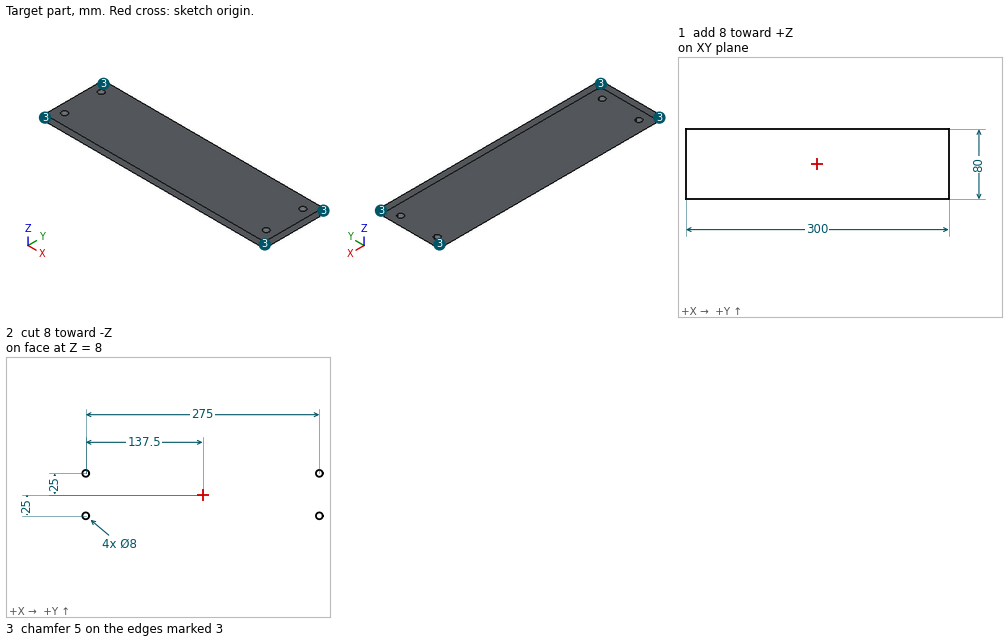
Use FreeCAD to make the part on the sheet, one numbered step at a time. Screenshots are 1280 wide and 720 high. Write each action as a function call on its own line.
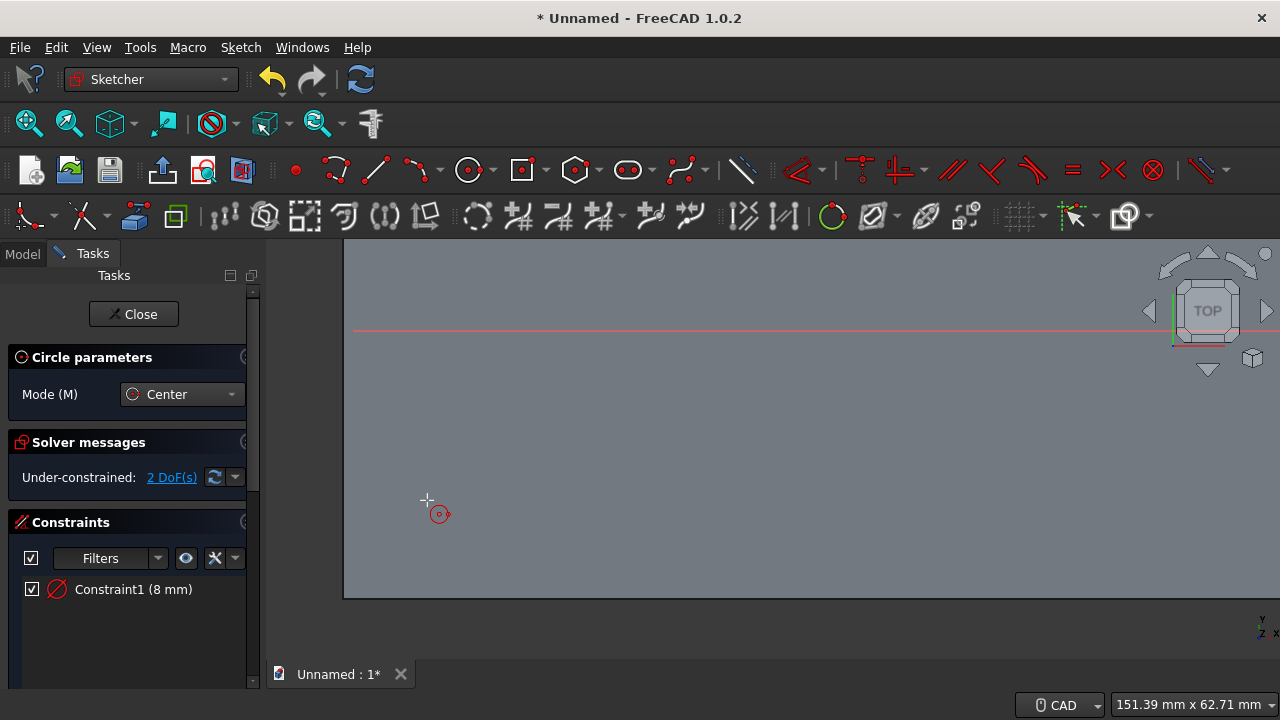
click(426, 498)
move(445, 479)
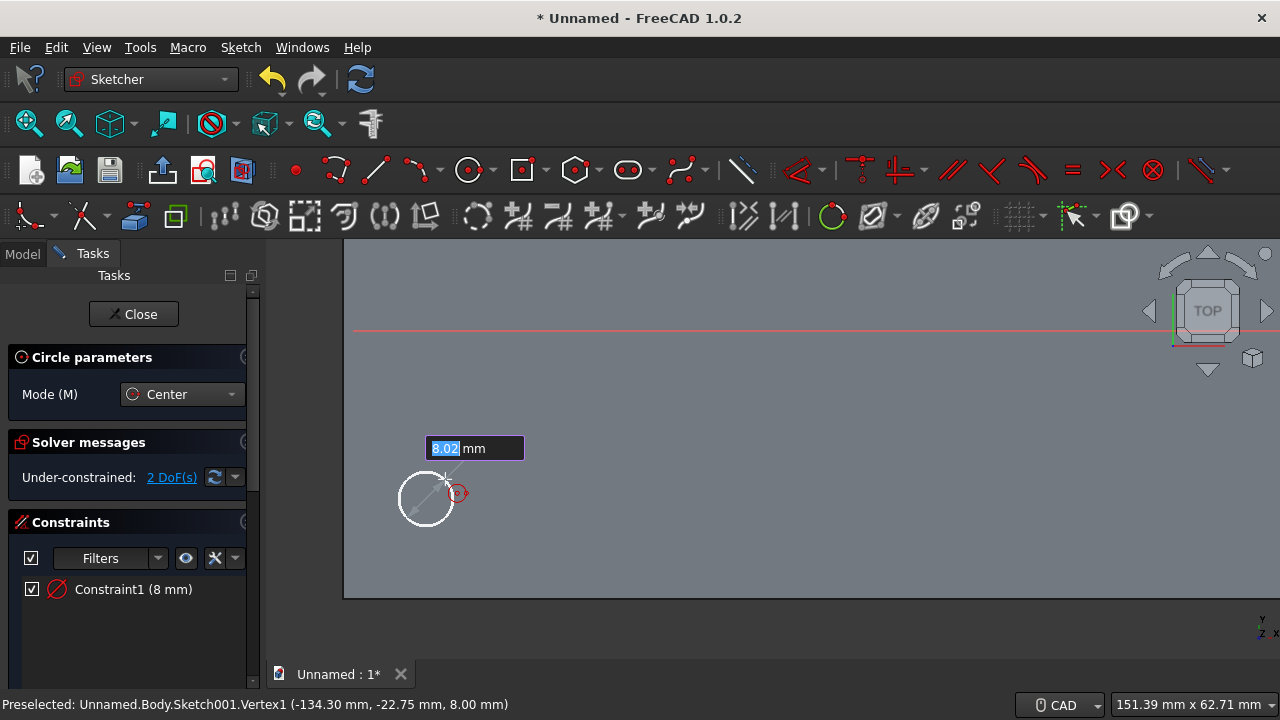
text(8)
key(Return)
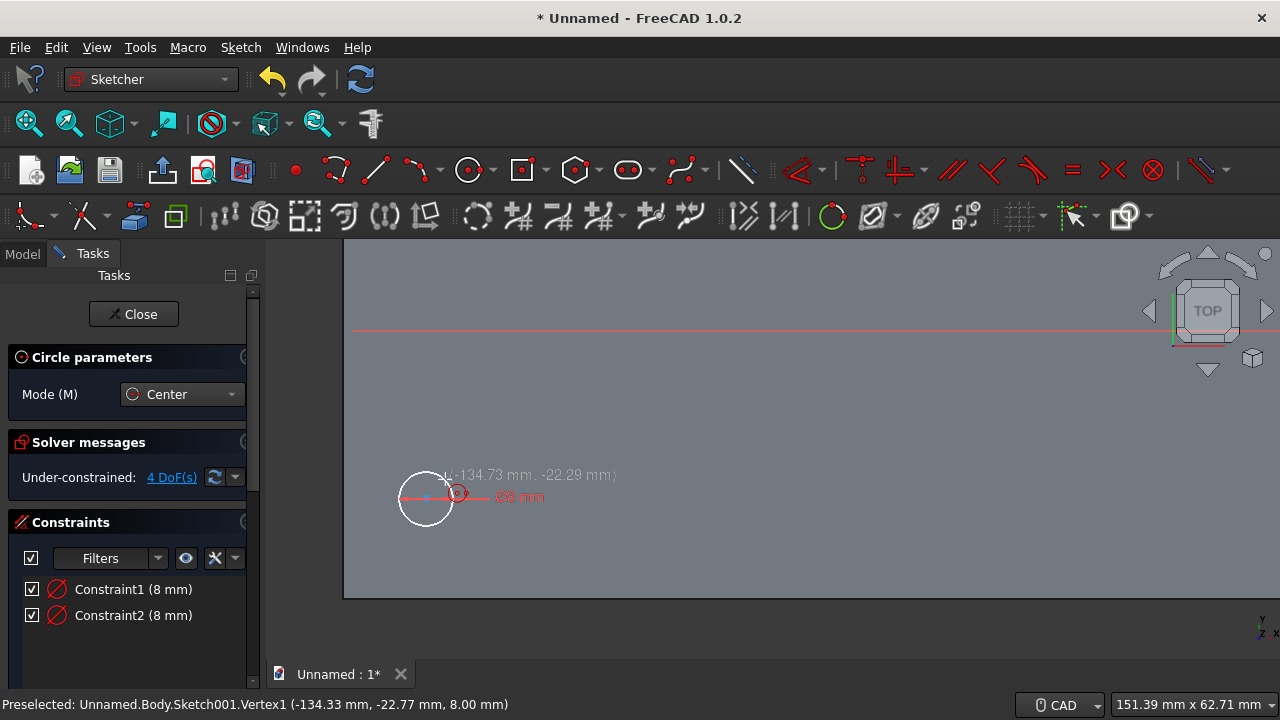
scroll(427, 500, down, 6)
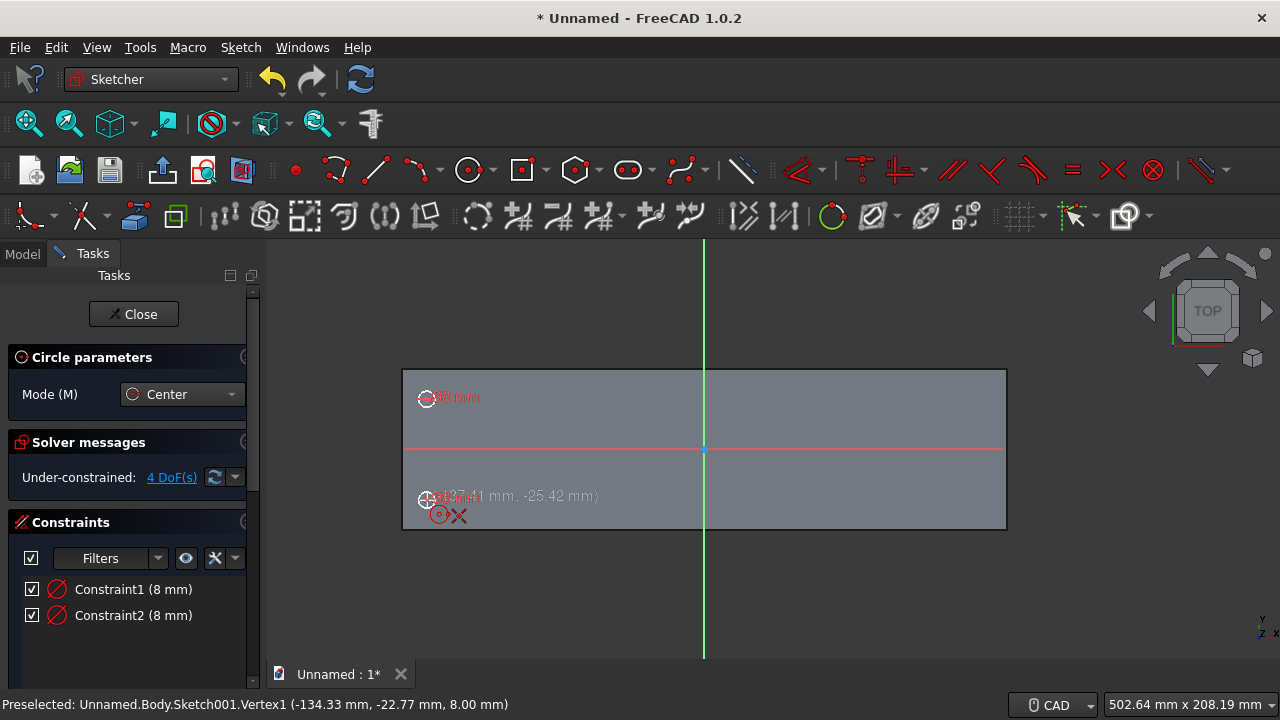
scroll(982, 399, up, 6)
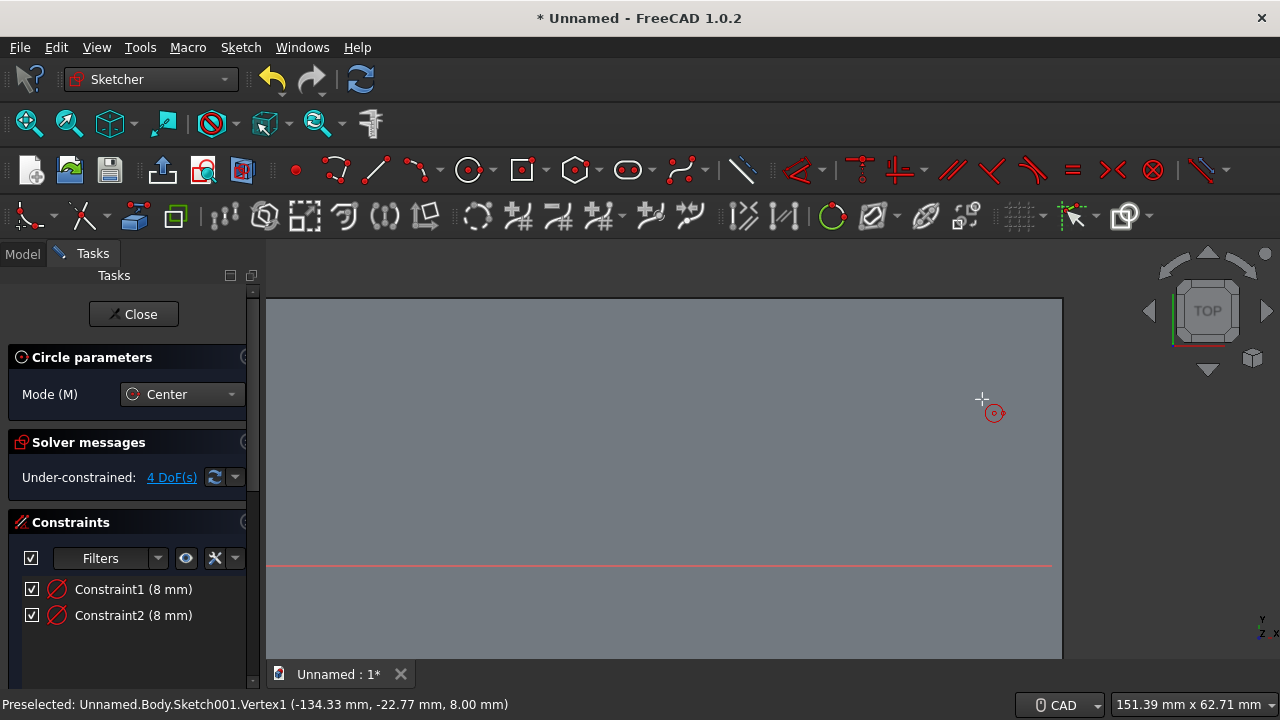
click(979, 398)
move(998, 379)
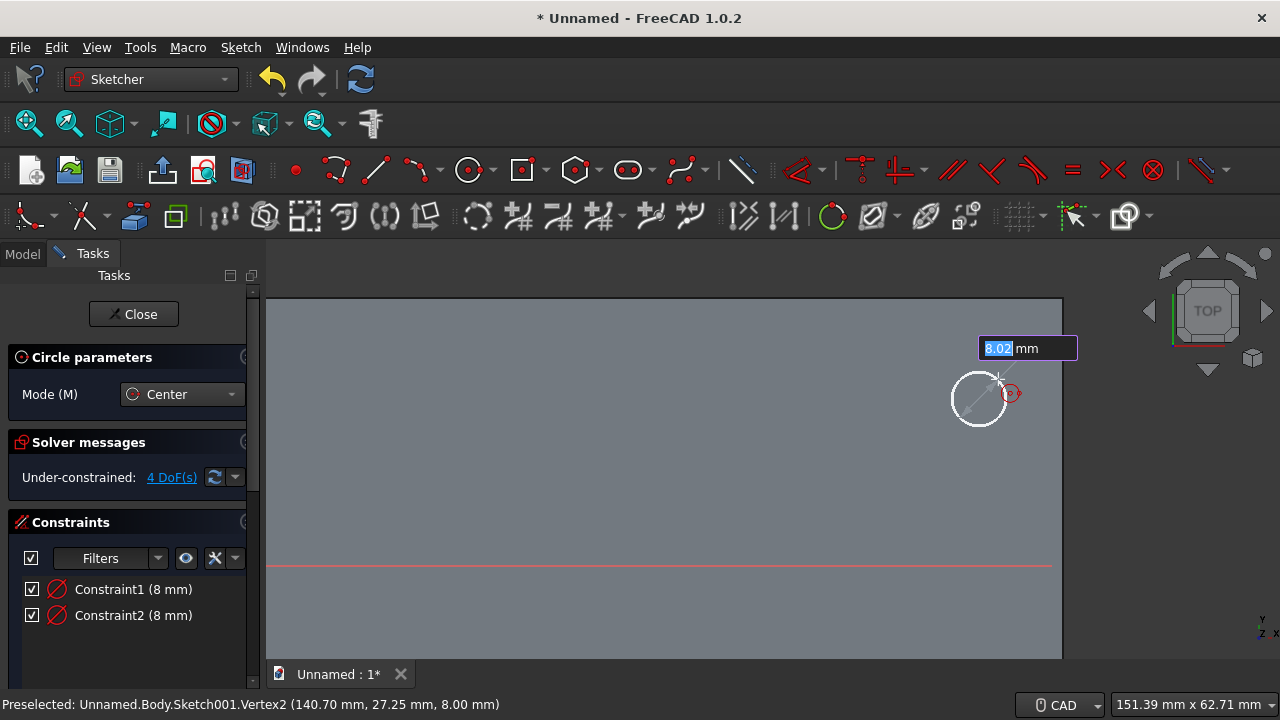
text(8)
key(Return)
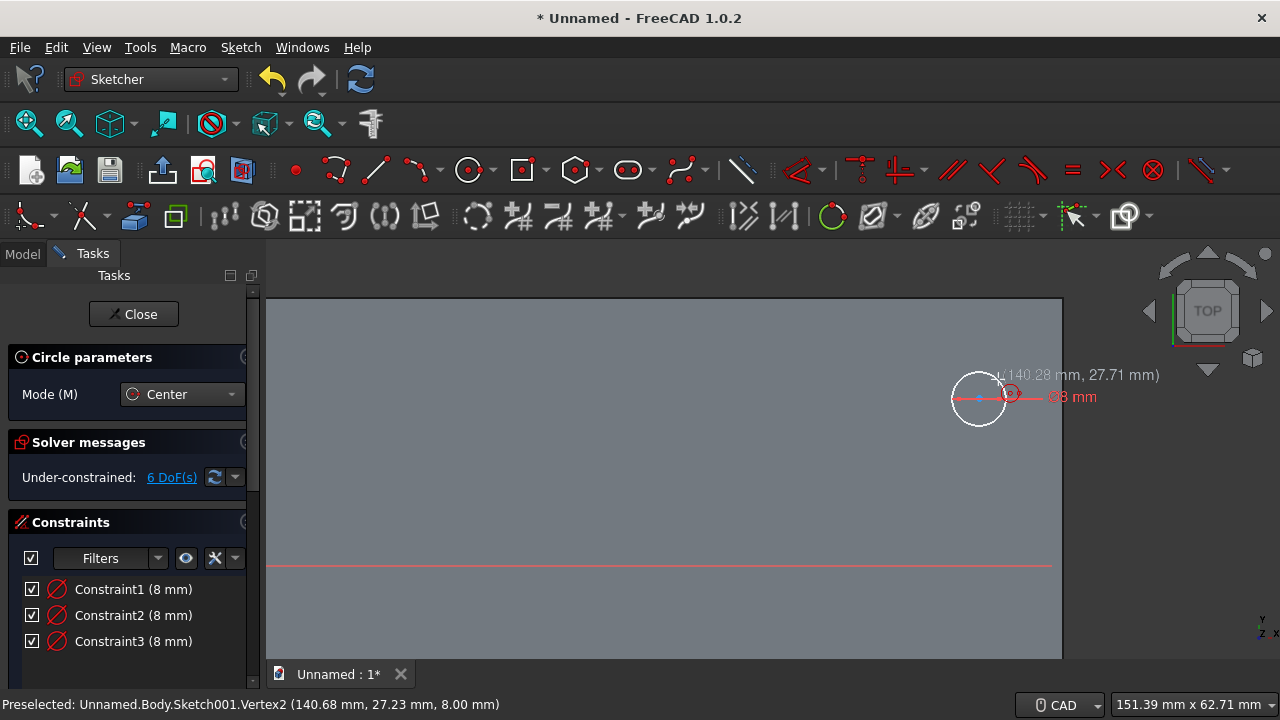
scroll(983, 399, down, 6)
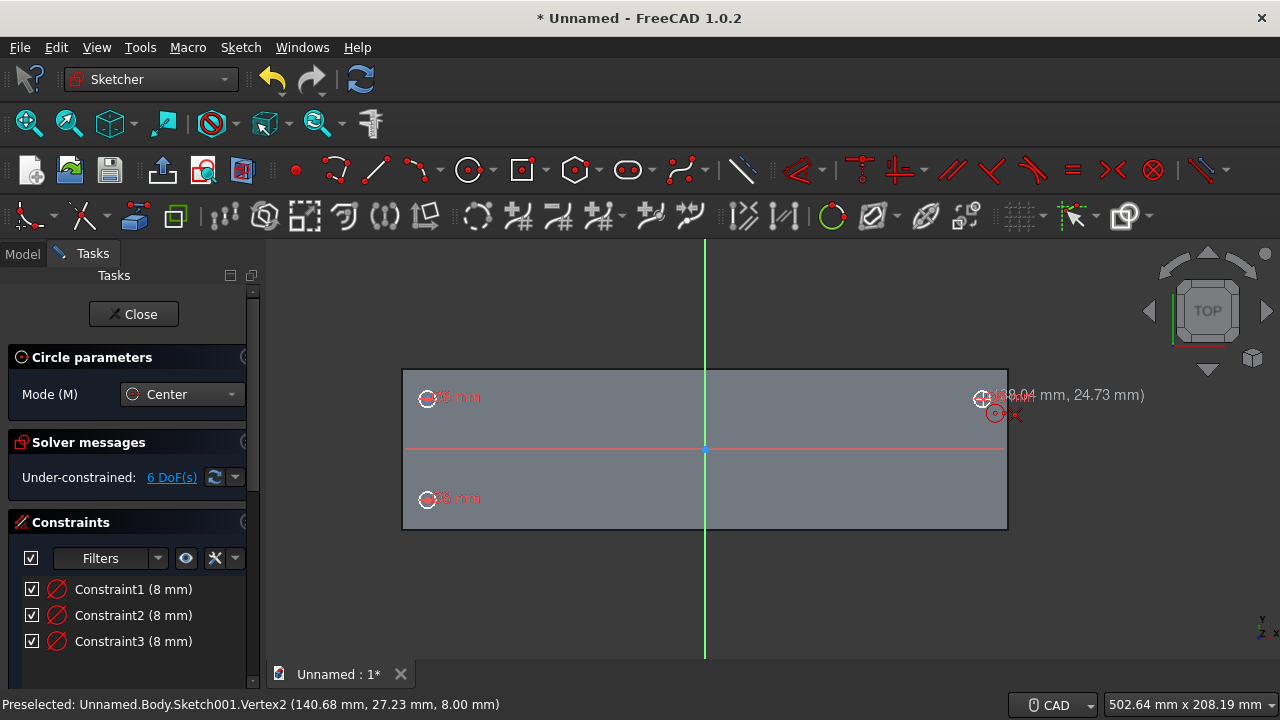
scroll(982, 500, up, 6)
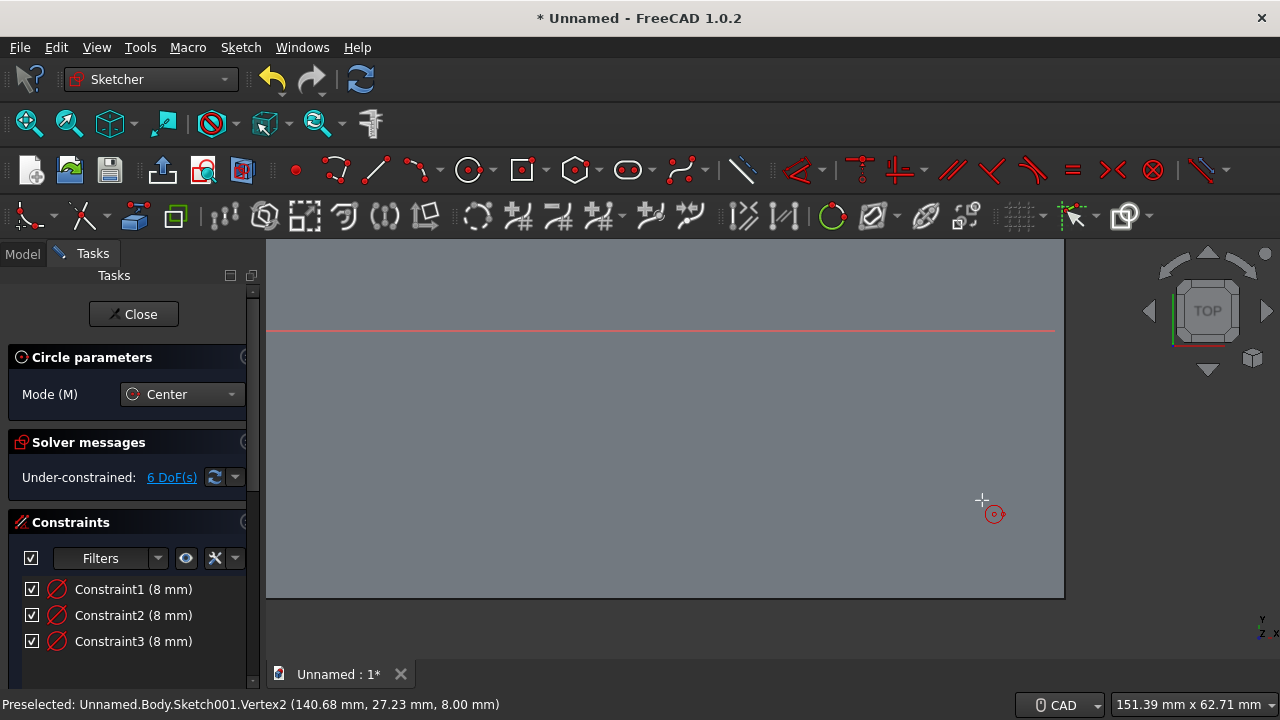
click(982, 498)
move(1001, 479)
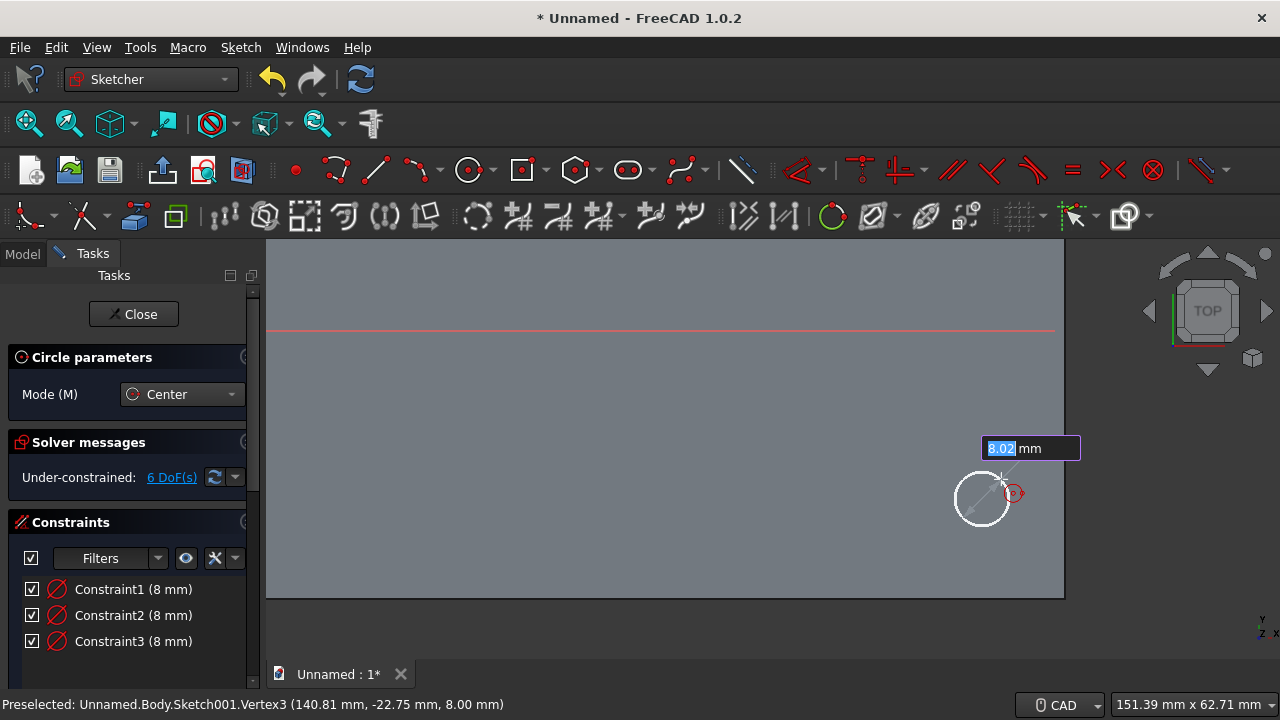
text(8)
key(Return)
key(Escape)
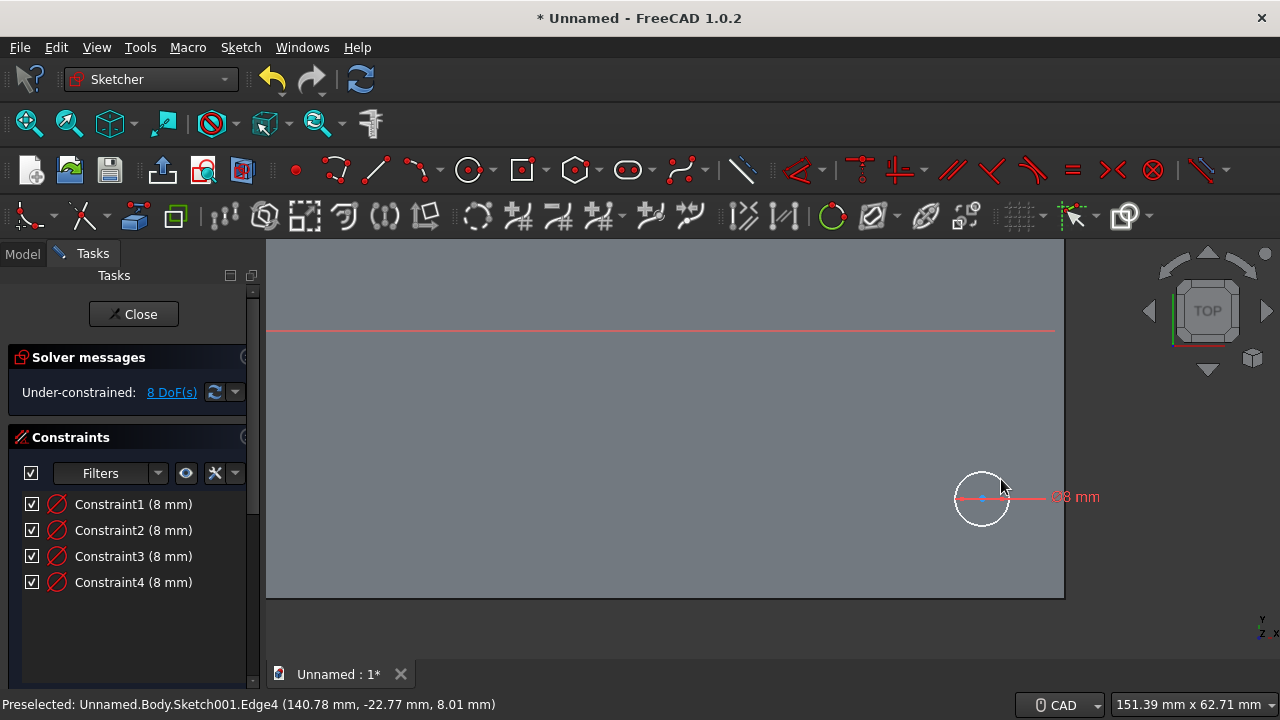
scroll(982, 500, down, 6)